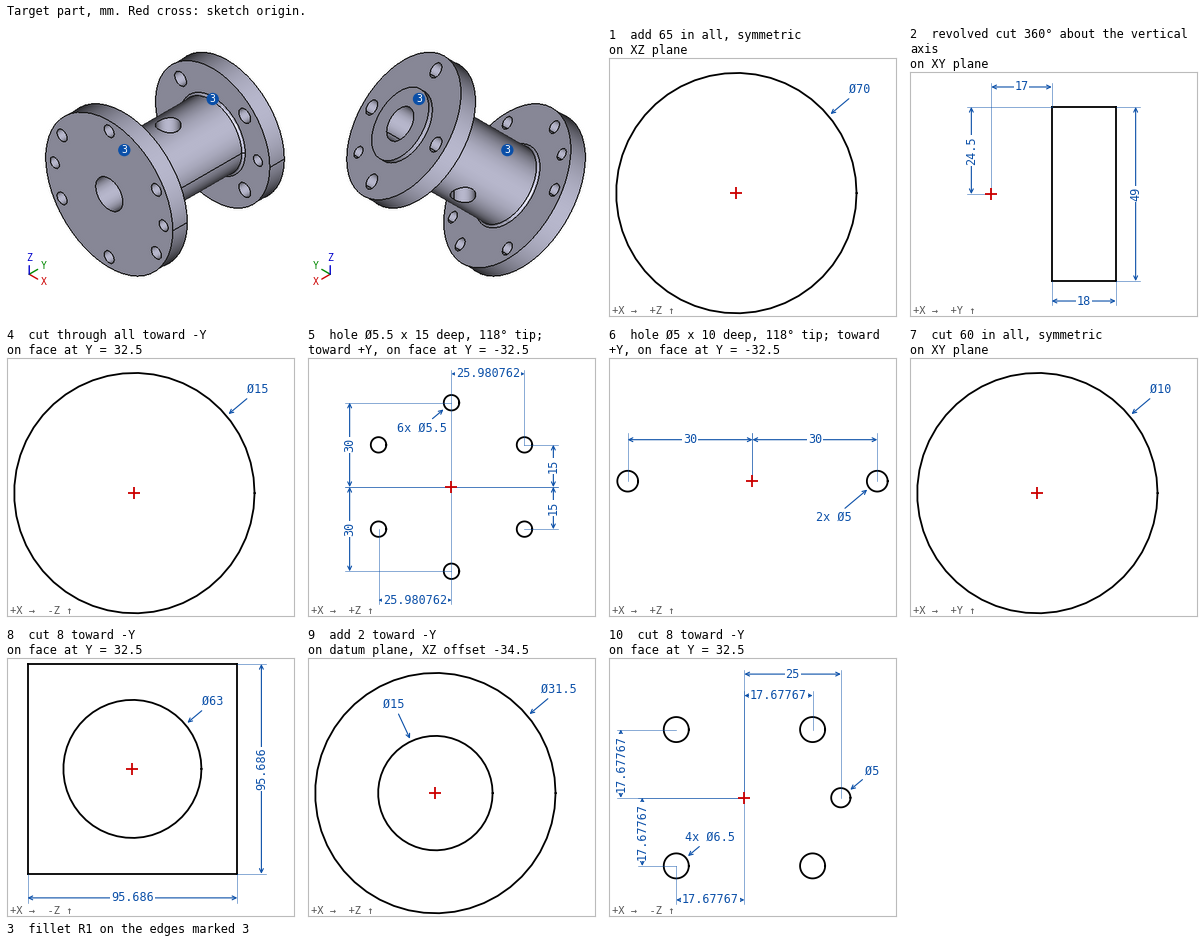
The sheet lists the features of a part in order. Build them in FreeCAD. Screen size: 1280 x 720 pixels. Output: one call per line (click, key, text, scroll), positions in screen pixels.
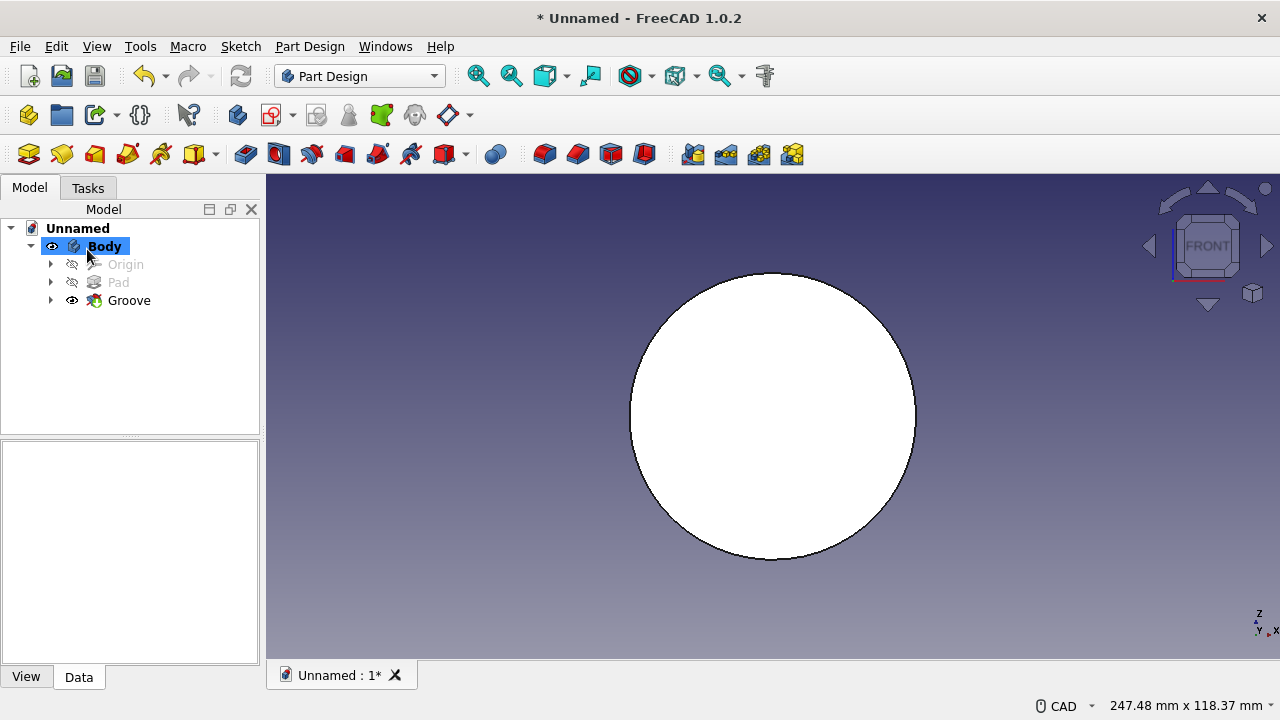
key(3)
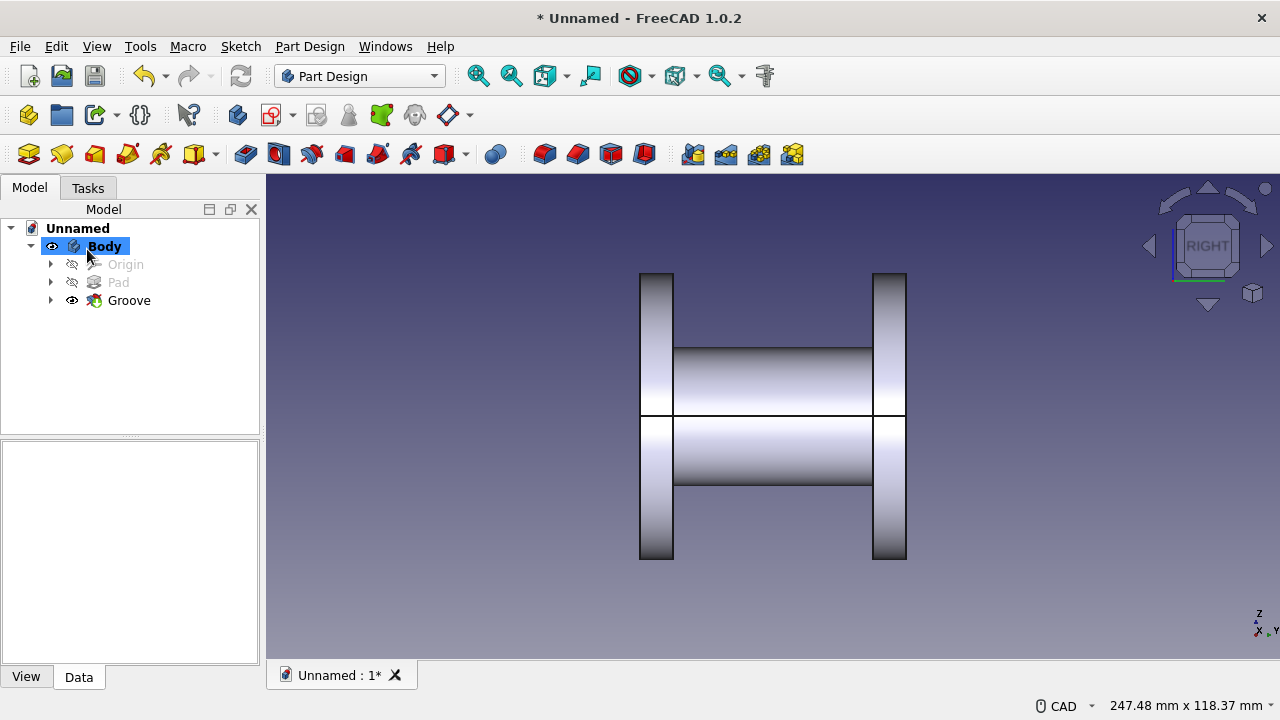
key(5)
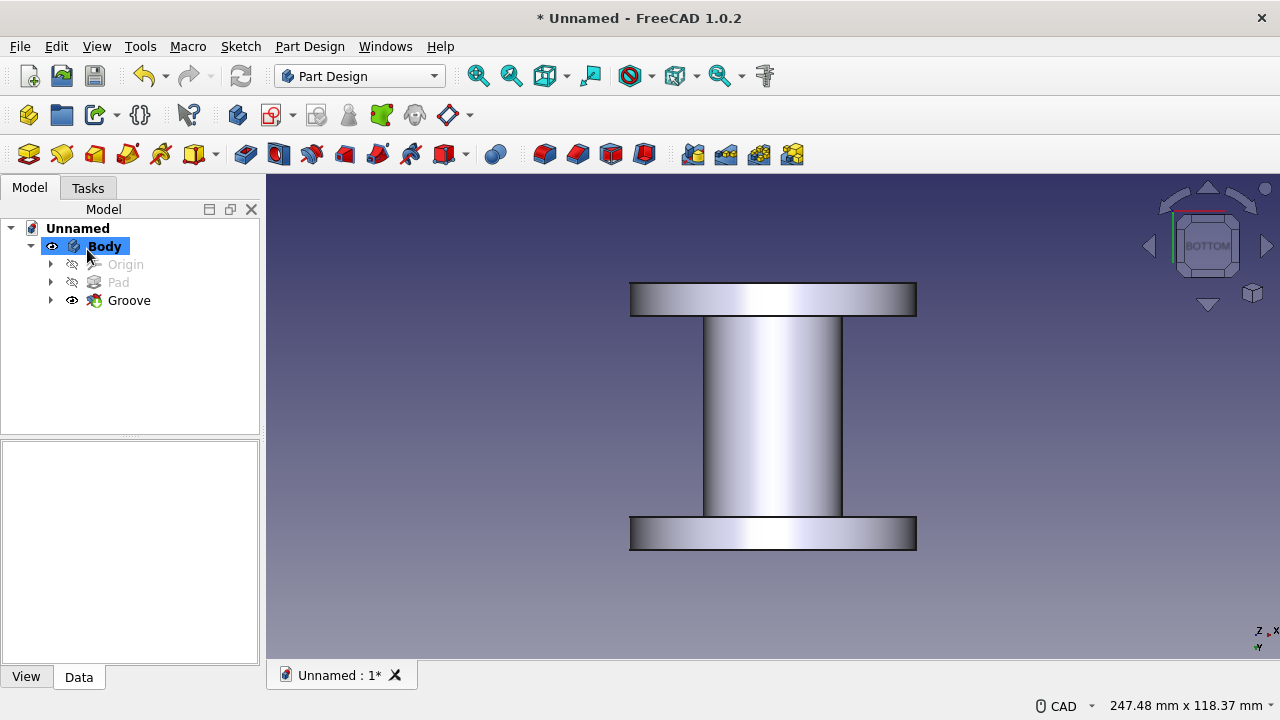
key(4)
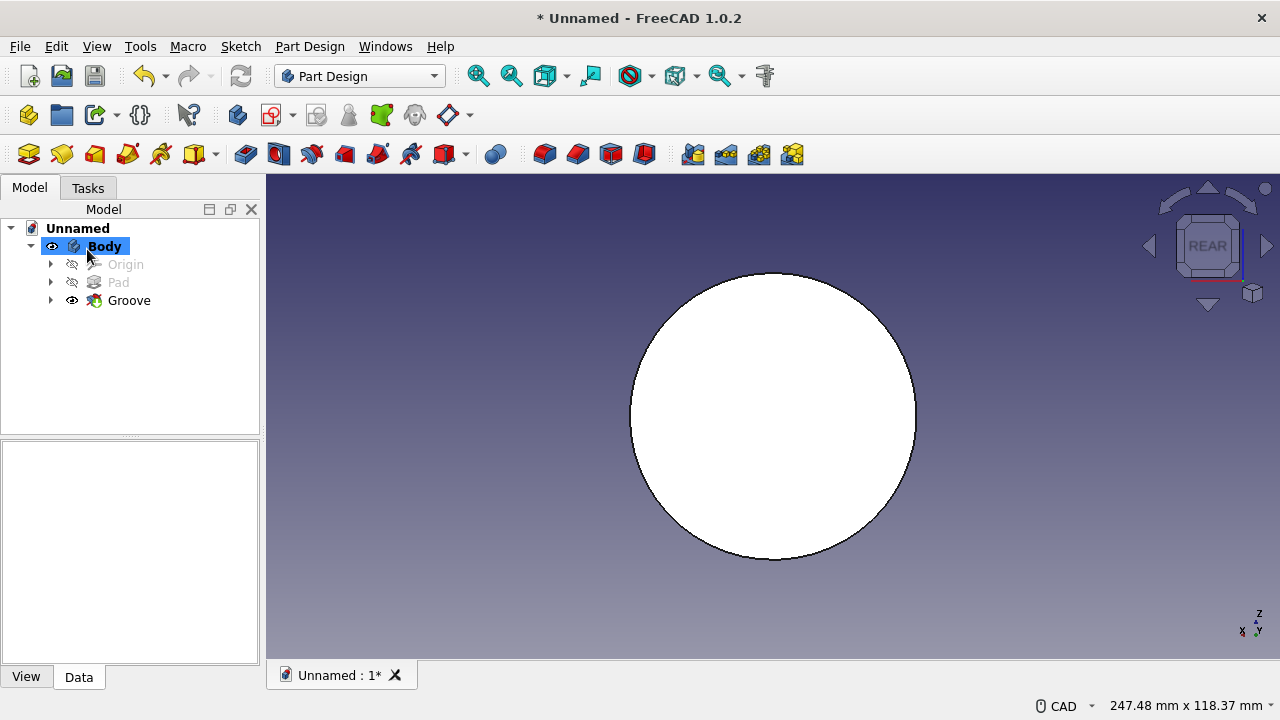
key(6)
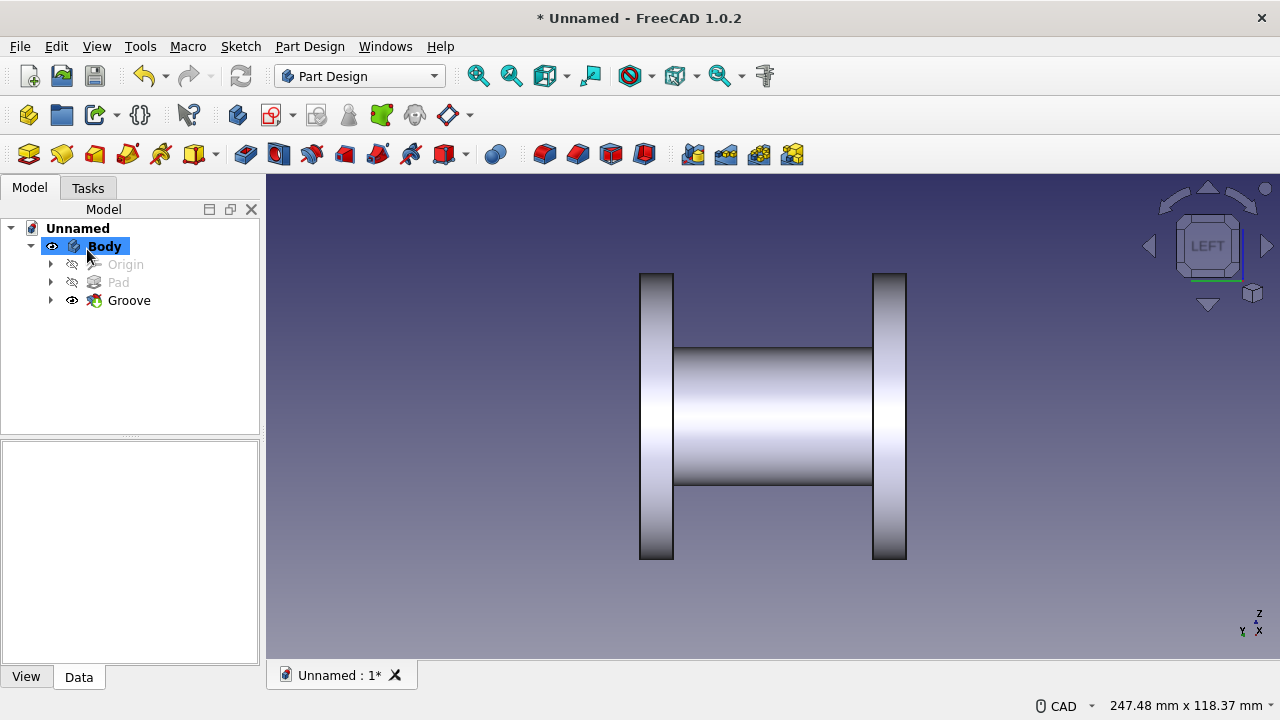
key(v)
key(3)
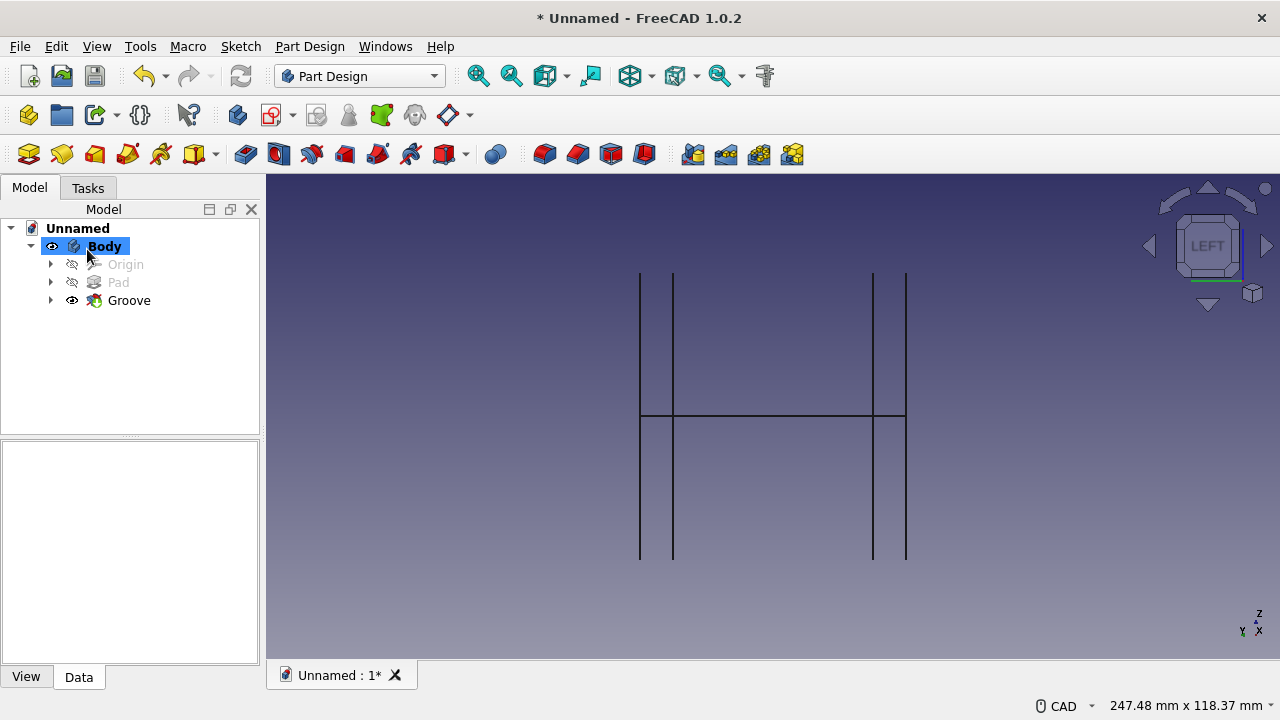
key(0)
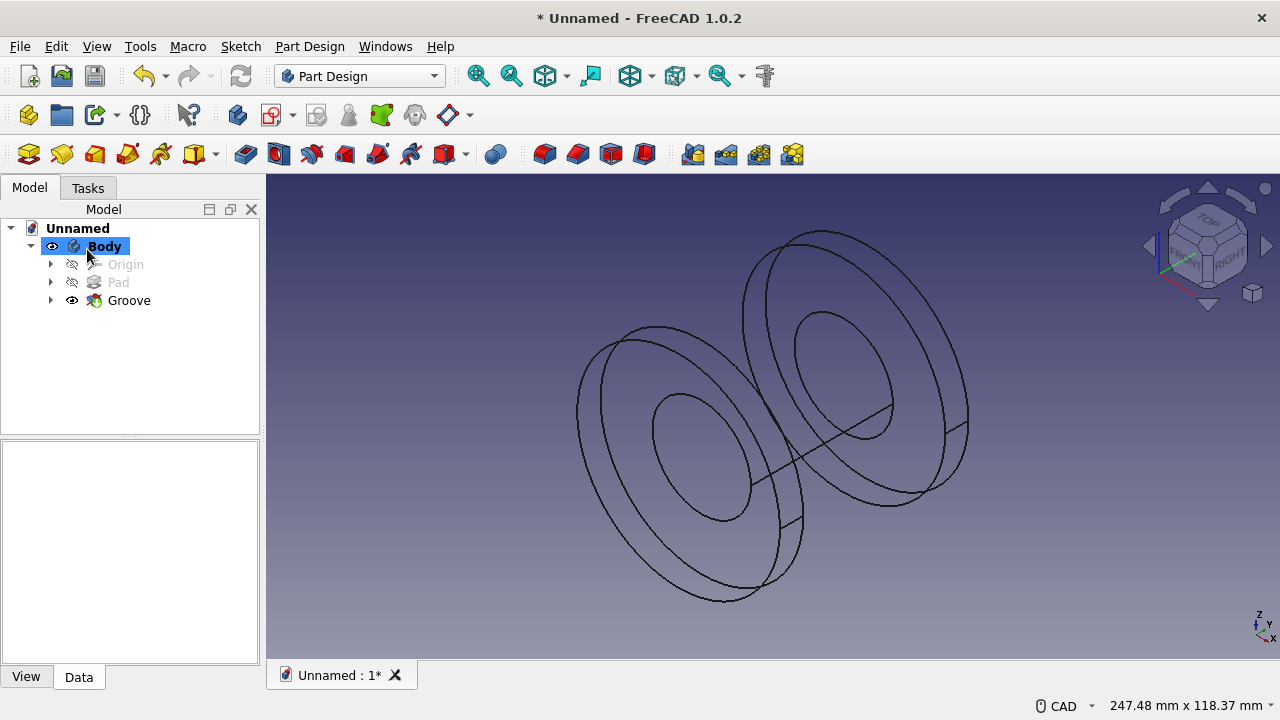
click(795, 346)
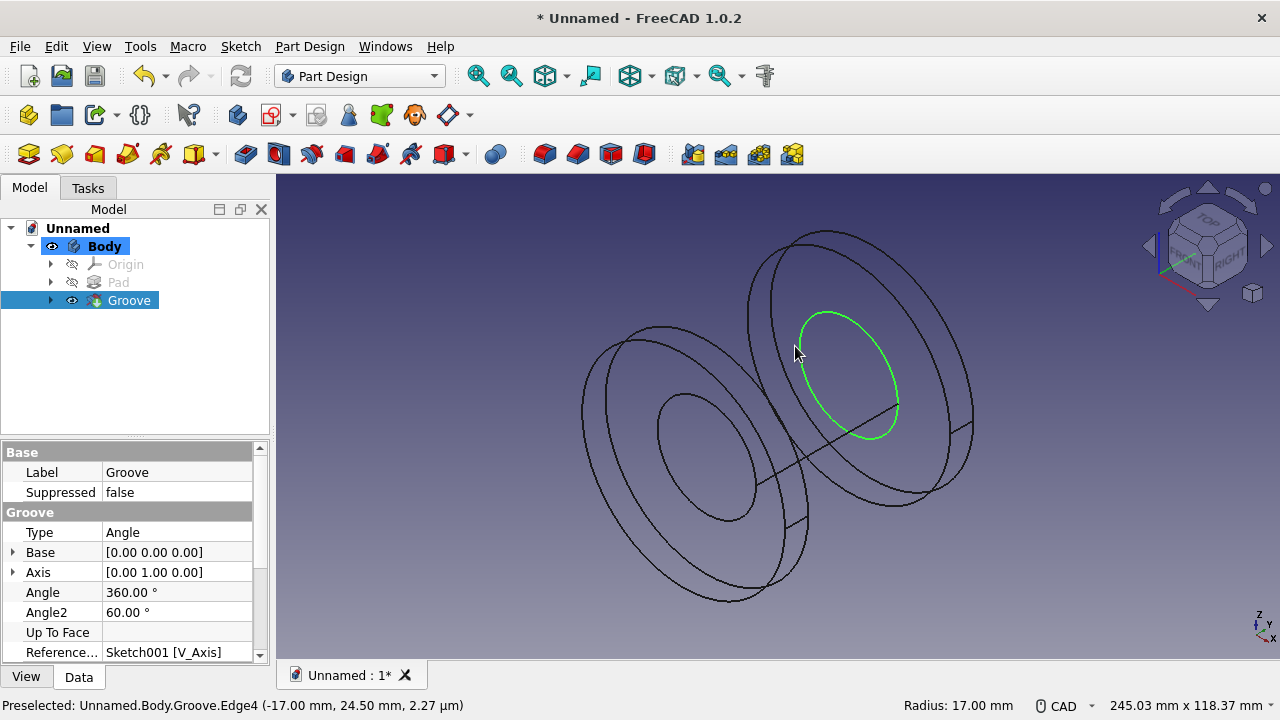
click(658, 428, ctrl)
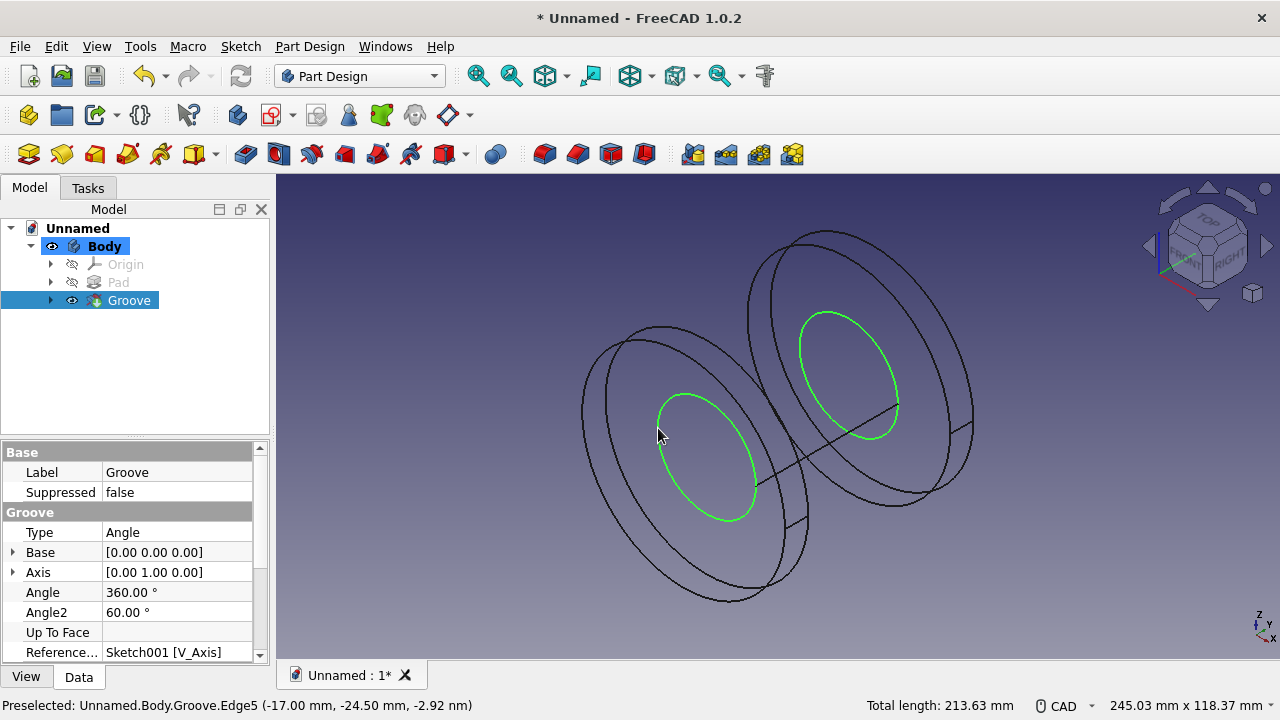
key(v)
key(1)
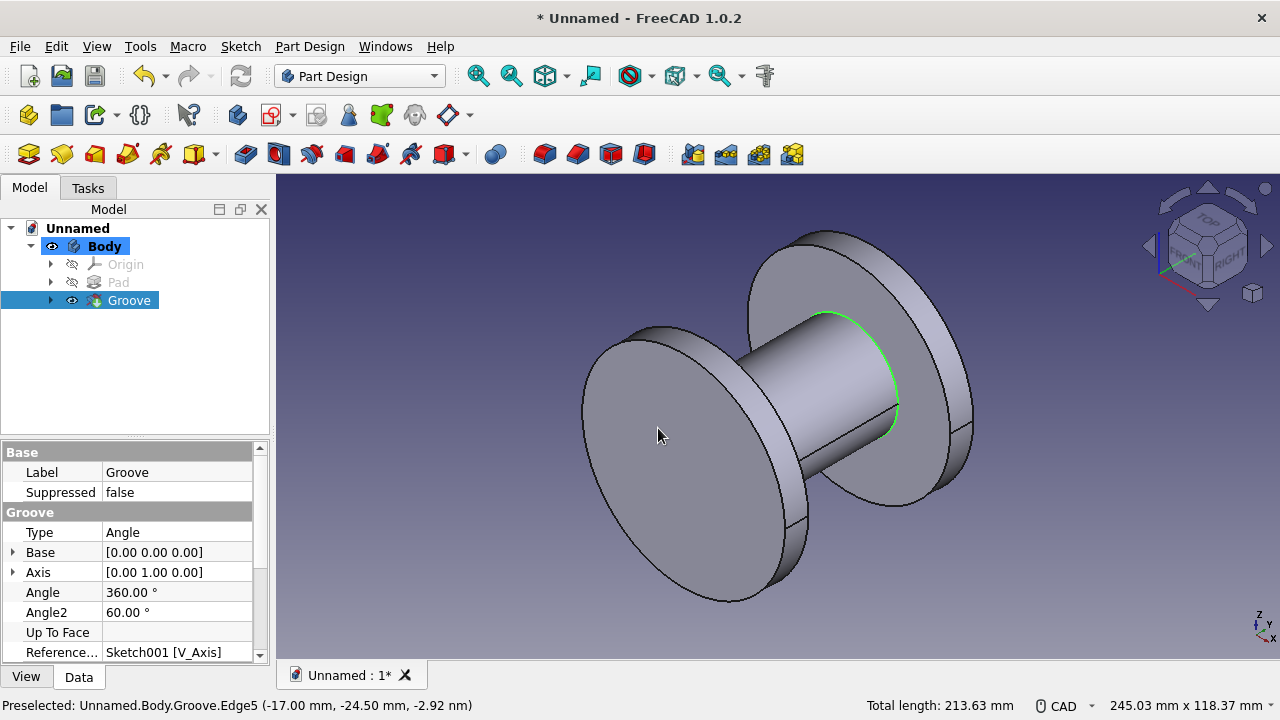
click(545, 154)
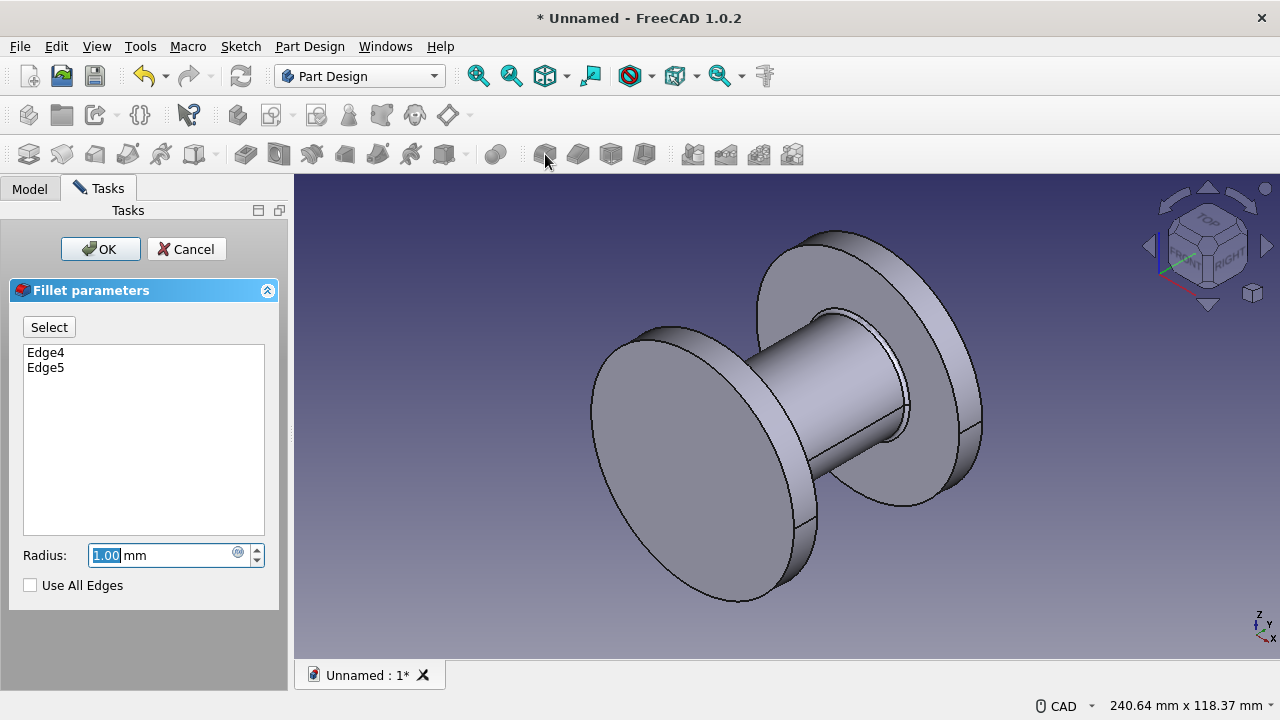
text(1)
key(Tab)